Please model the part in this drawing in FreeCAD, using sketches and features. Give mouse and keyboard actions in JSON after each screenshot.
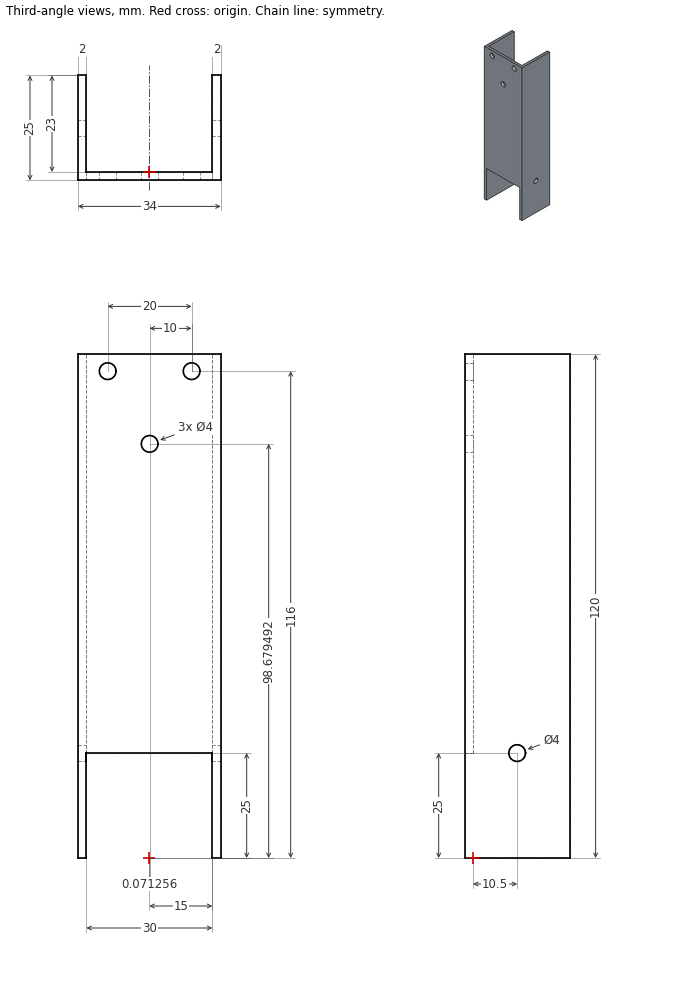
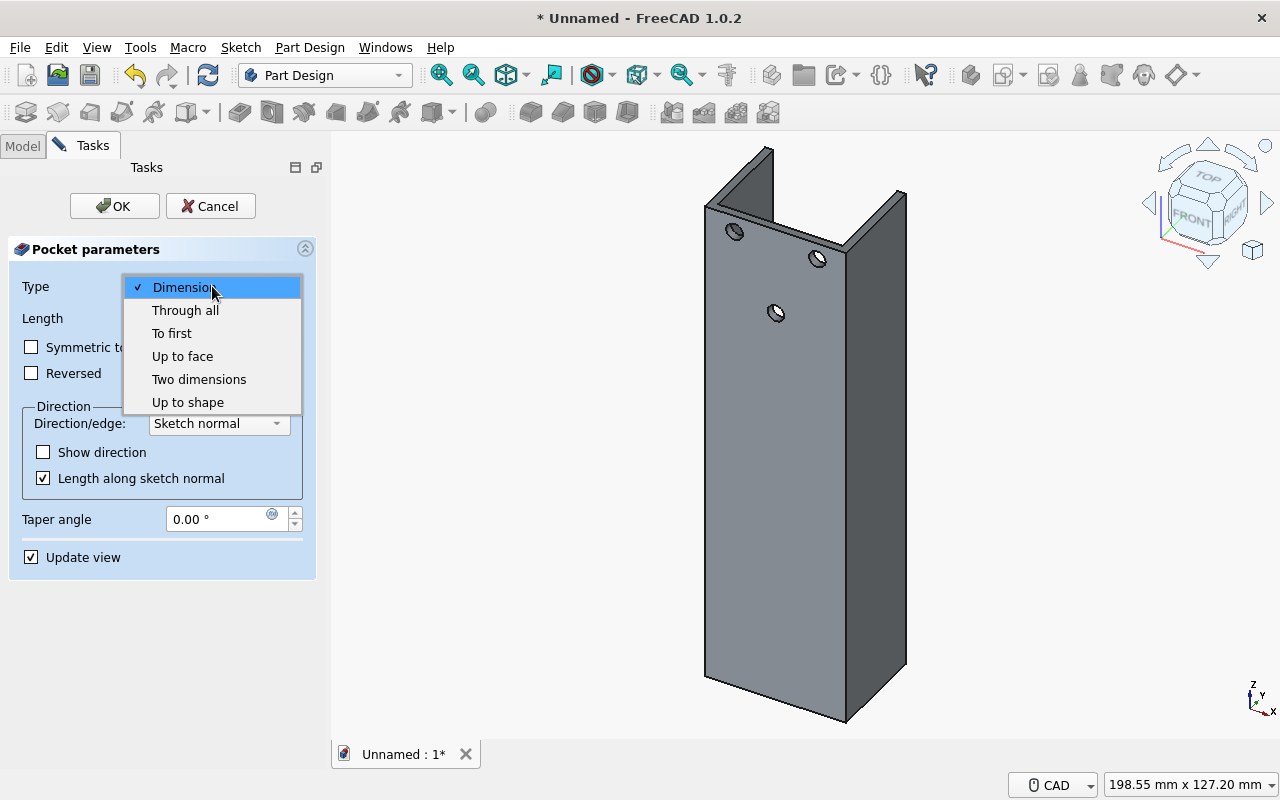
{"action": "left_click", "coordinate": [212, 310]}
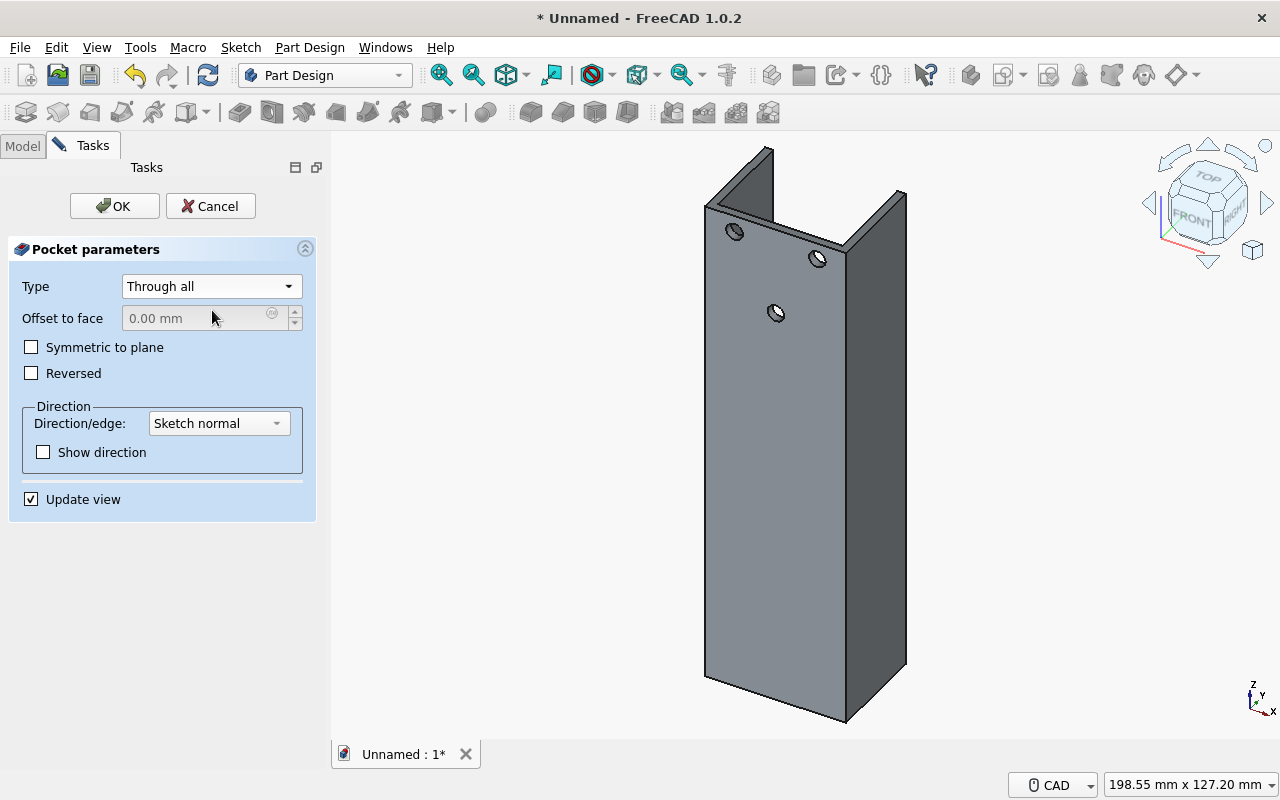
{"action": "left_click", "coordinate": [115, 206]}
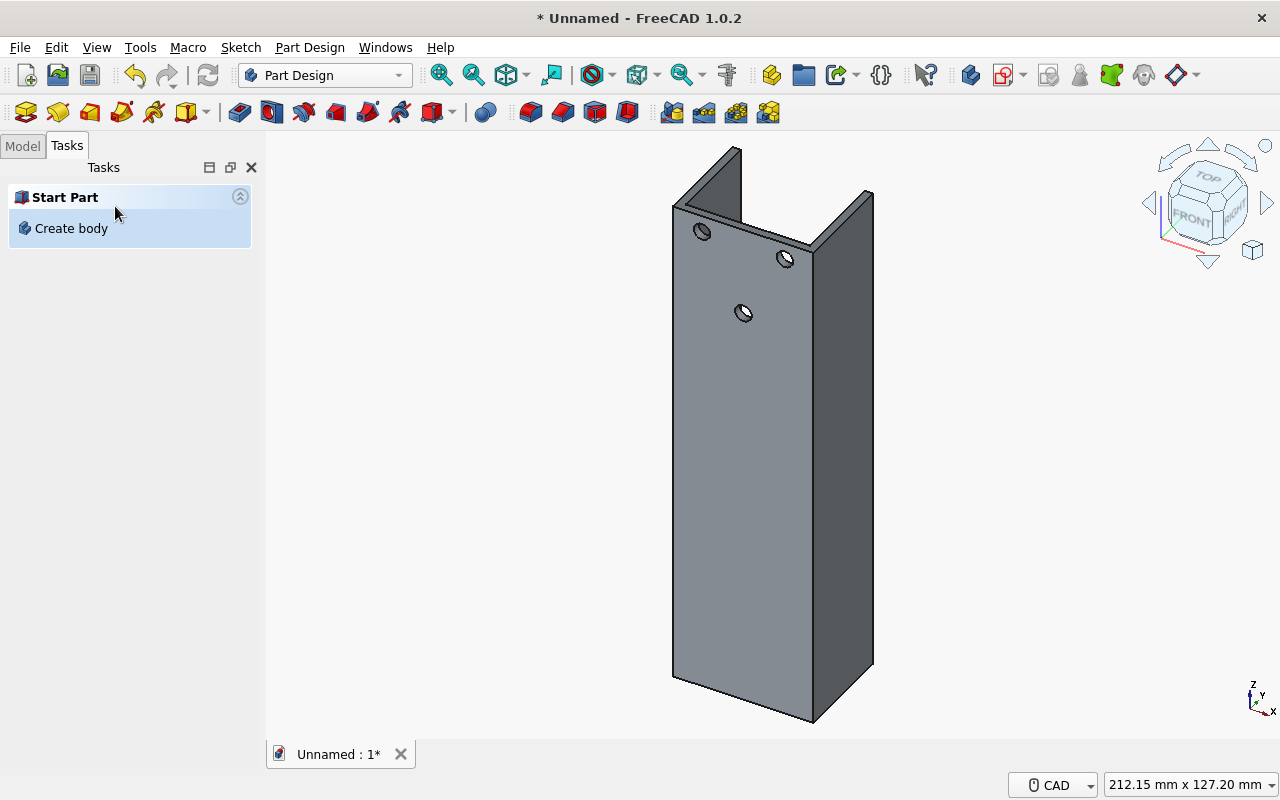
{"action": "key", "text": "4"}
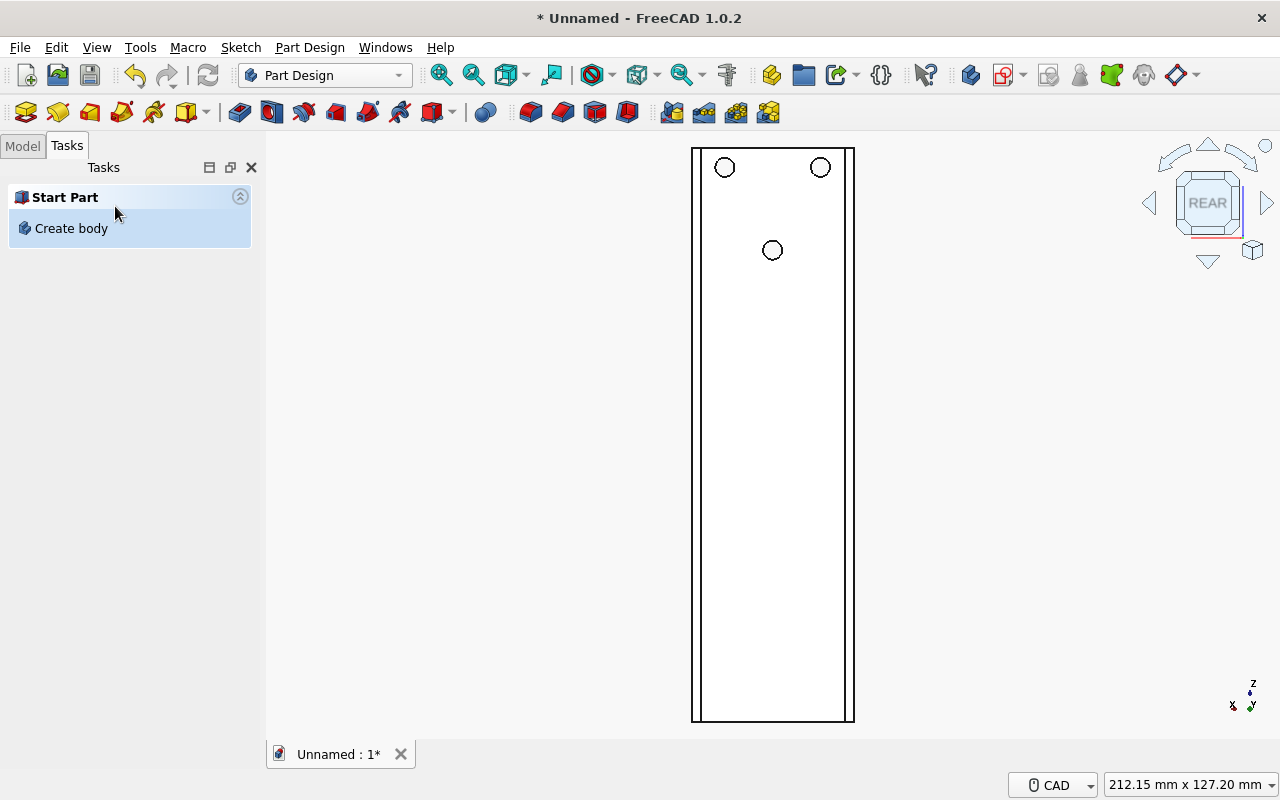
{"action": "left_click", "coordinate": [773, 352]}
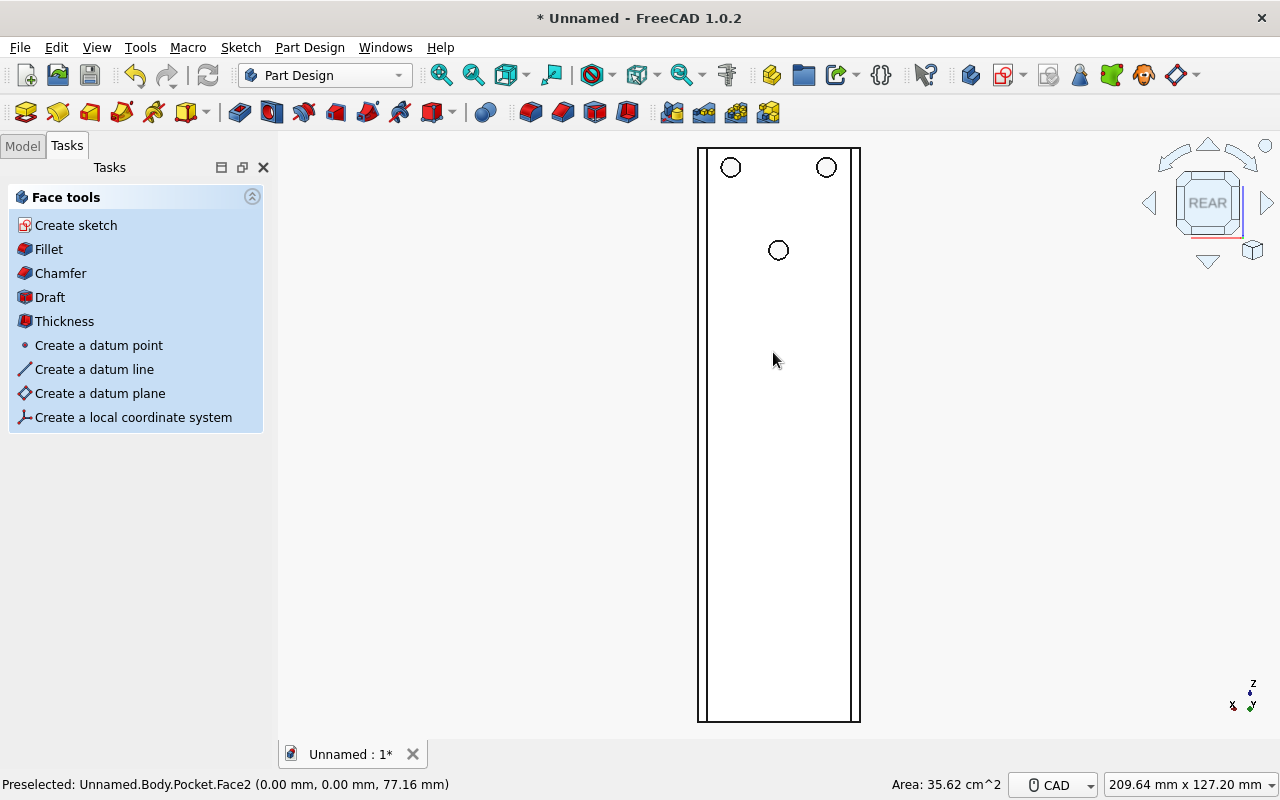
{"action": "left_click", "coordinate": [1004, 76]}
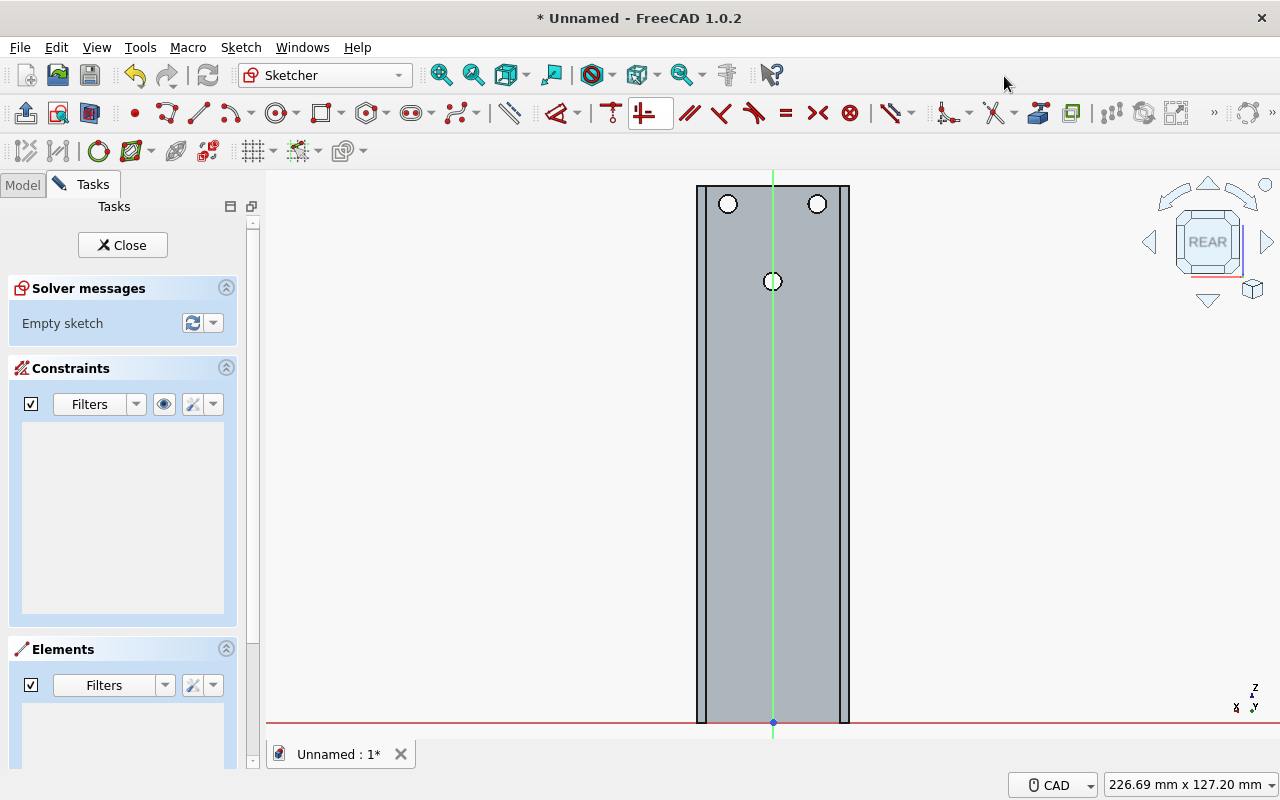
{"action": "left_click", "coordinate": [90, 114]}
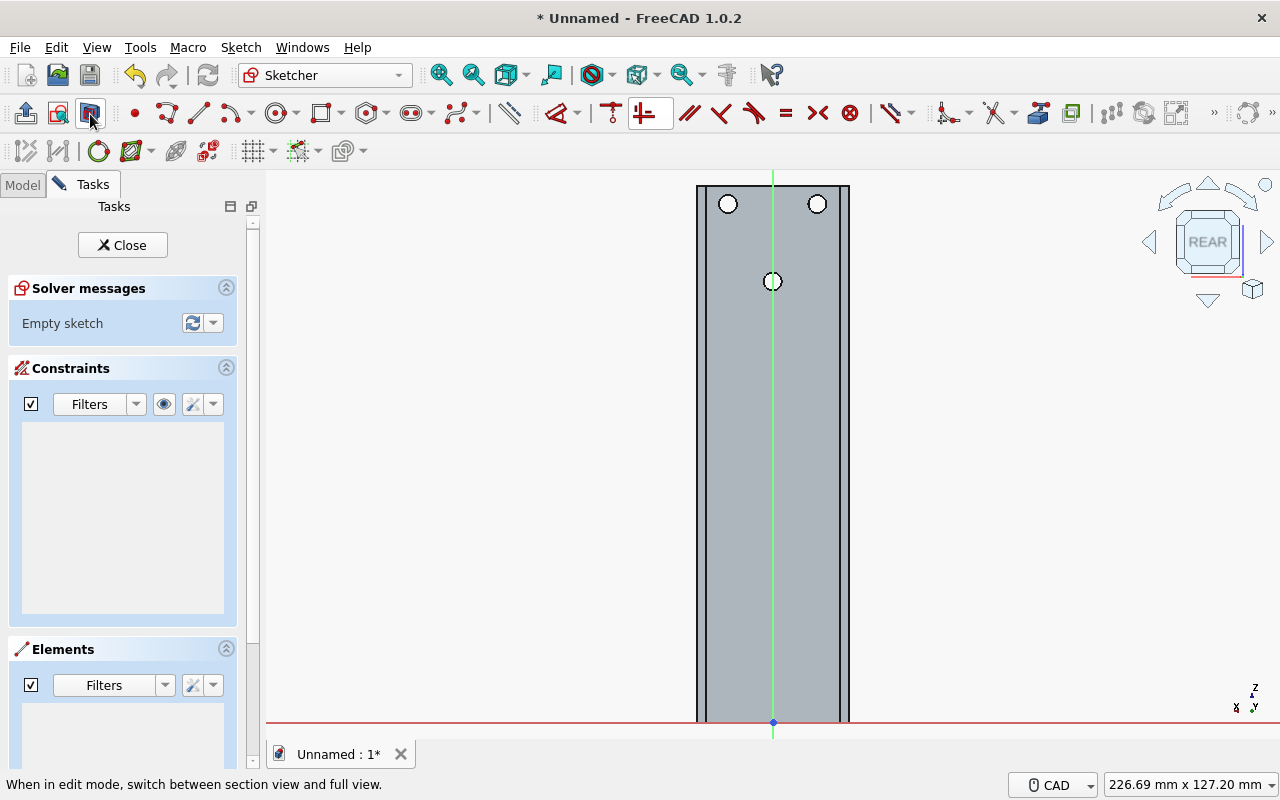
{"action": "scroll", "coordinate": [704, 454], "scroll_direction": "down", "scroll_amount": 5}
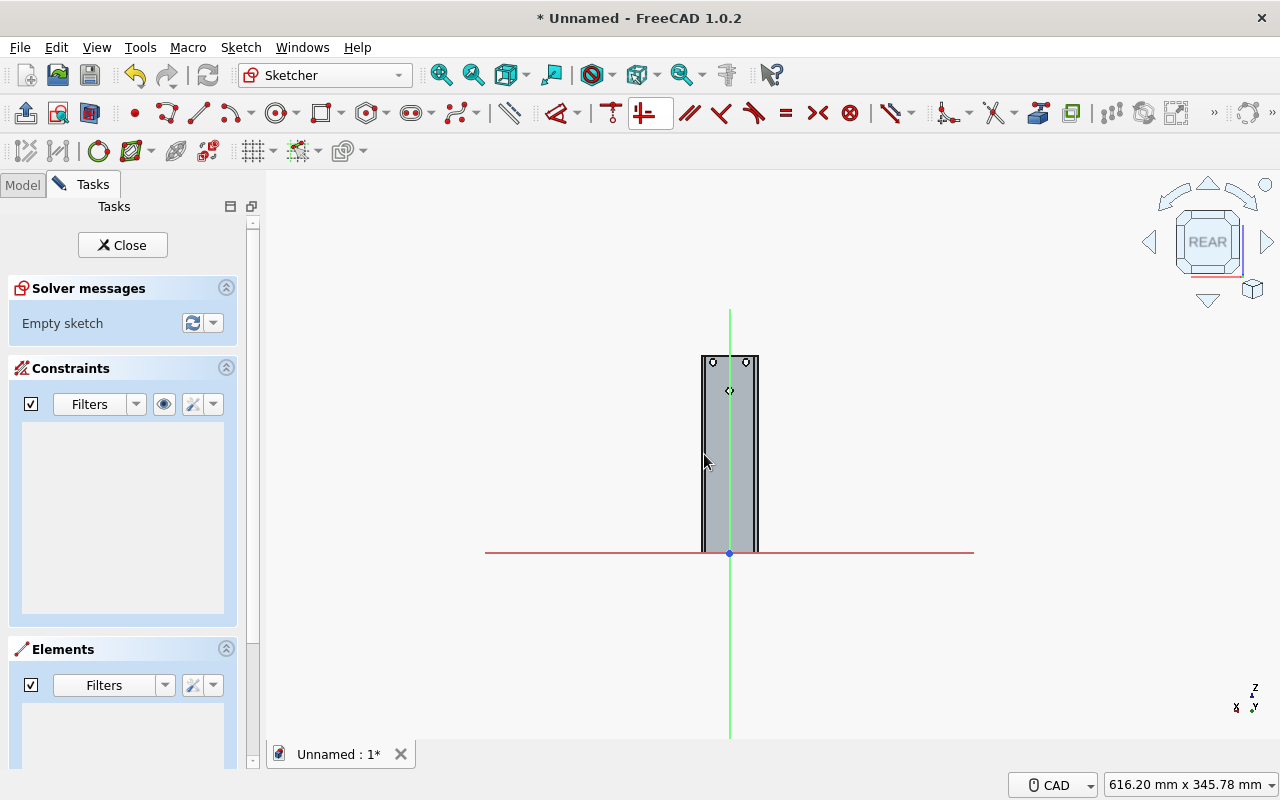
{"action": "scroll", "coordinate": [733, 542], "scroll_direction": "up", "scroll_amount": 11}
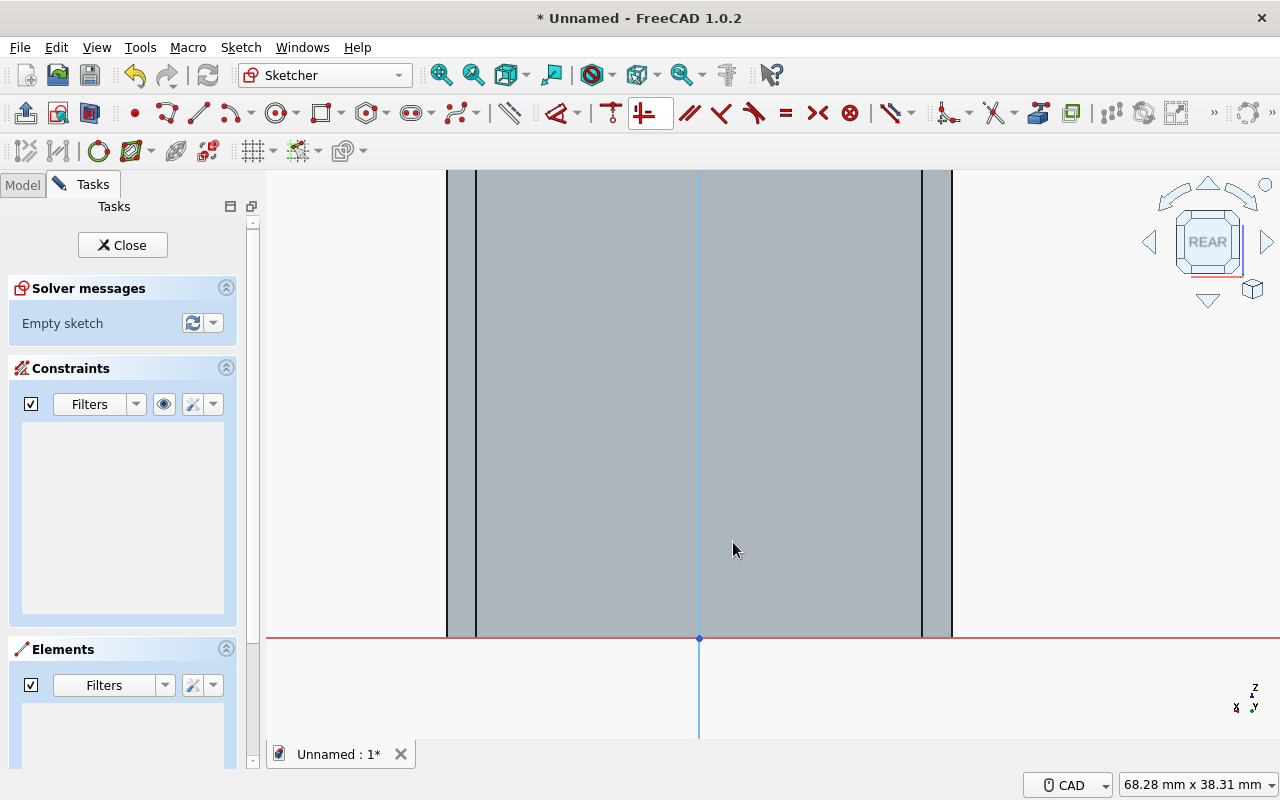
{"action": "left_click", "coordinate": [322, 114]}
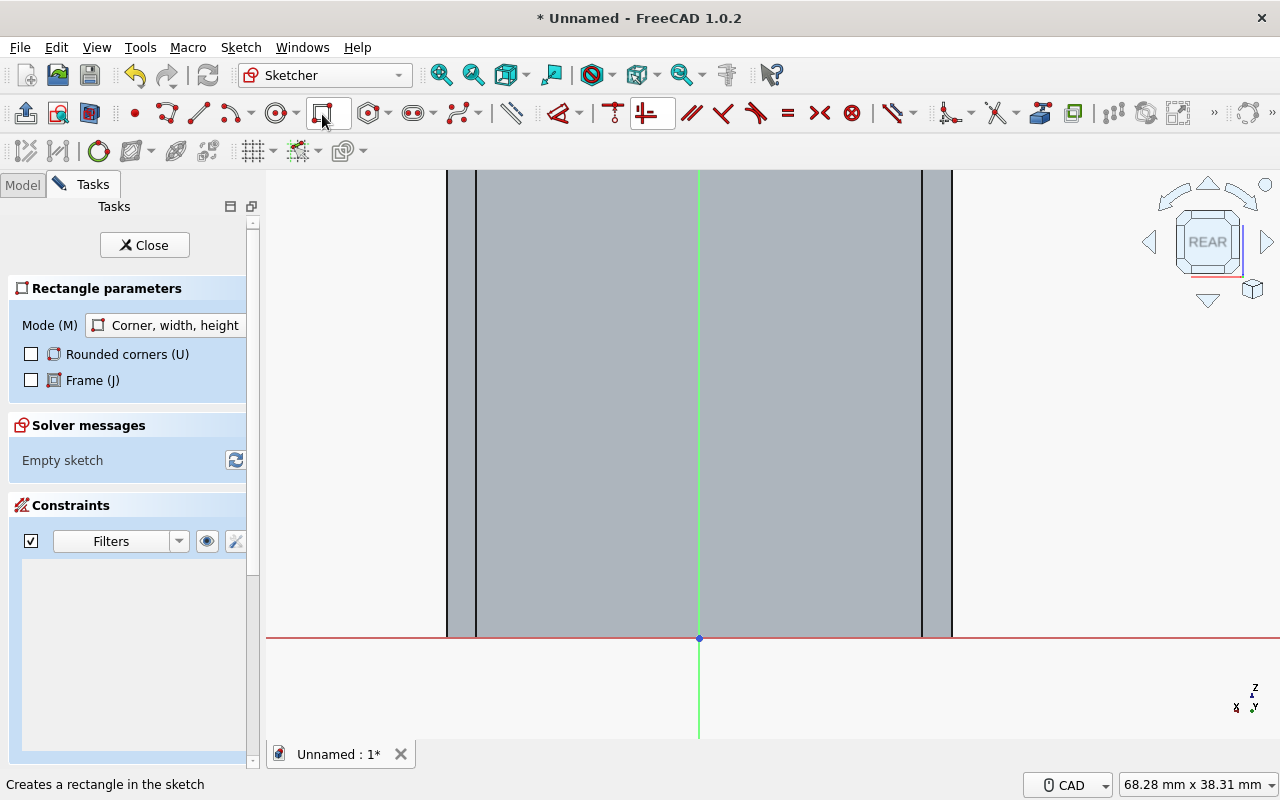
{"action": "left_click", "coordinate": [476, 267]}
{"action": "left_click", "coordinate": [922, 638]}
{"action": "key", "text": "Escape"}